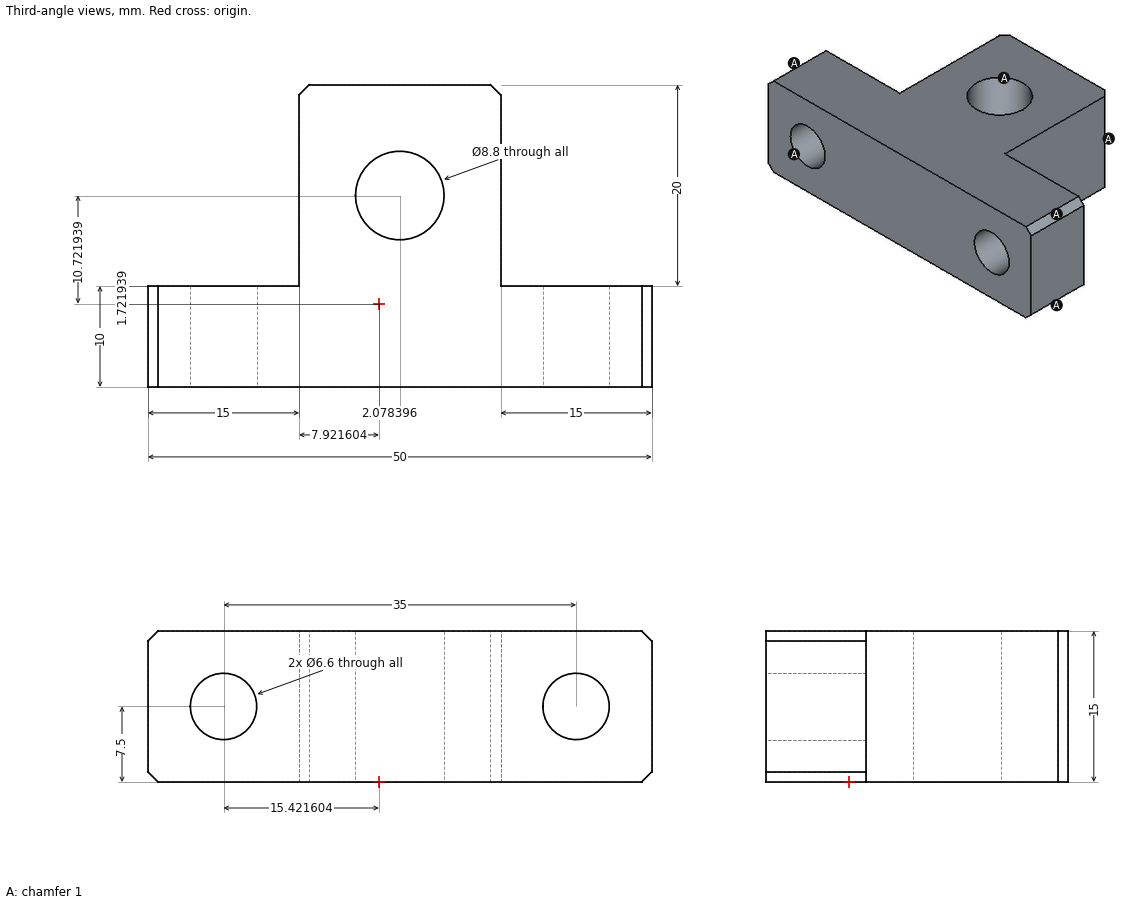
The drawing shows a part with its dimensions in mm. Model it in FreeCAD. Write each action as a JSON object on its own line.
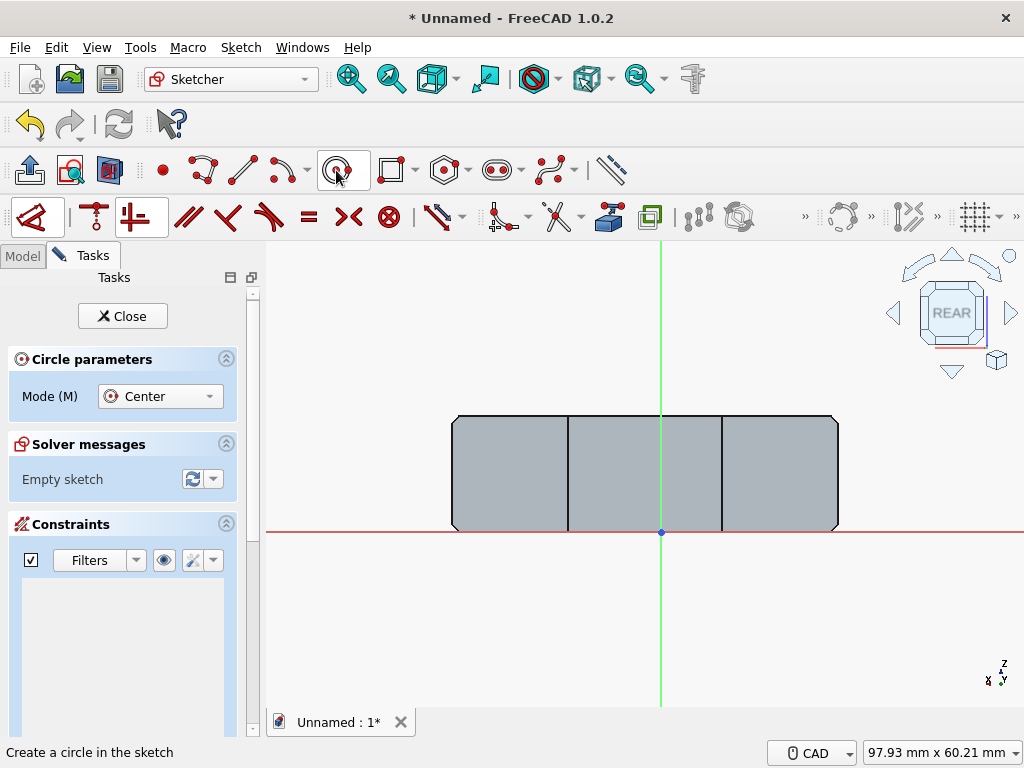
{"action": "left_click", "coordinate": [780, 474]}
{"action": "mouse_move", "coordinate": [799, 456]}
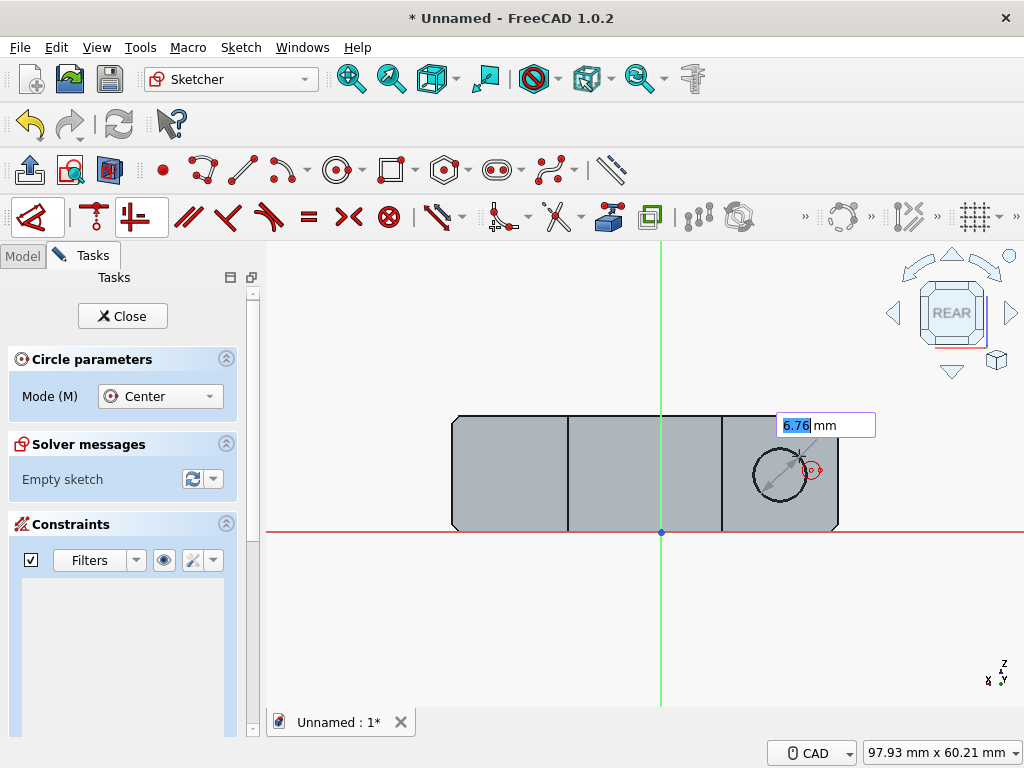
{"action": "type", "text": "6.6"}
{"action": "key", "text": "Return"}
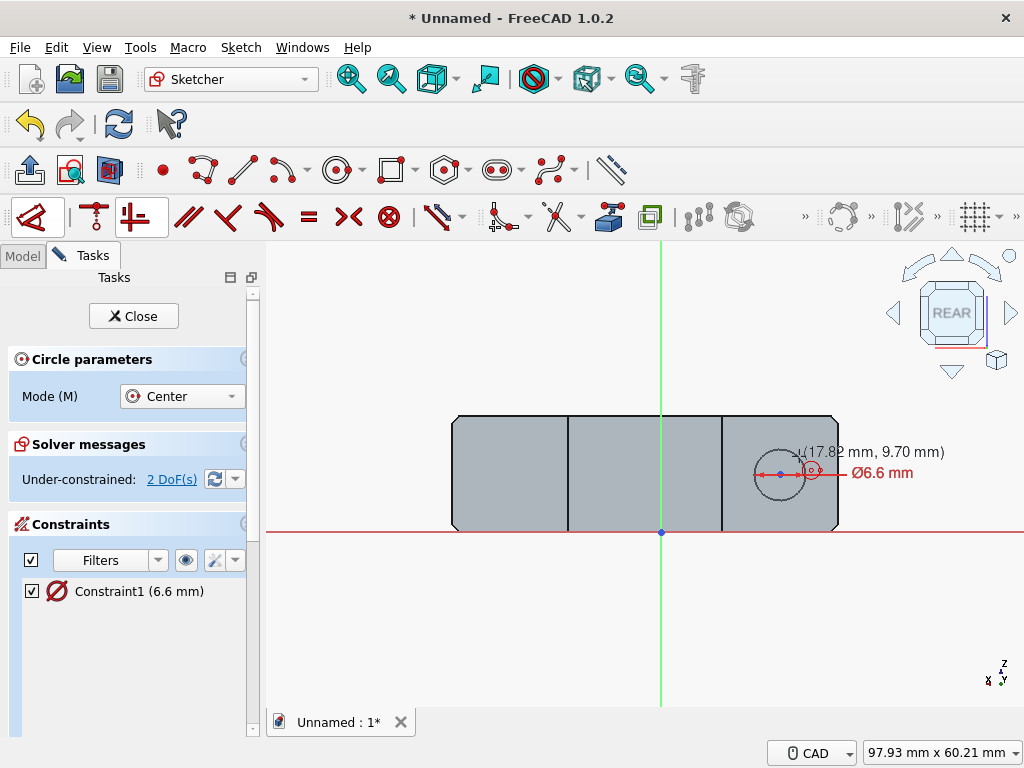
{"action": "left_click", "coordinate": [510, 474]}
{"action": "mouse_move", "coordinate": [528, 456]}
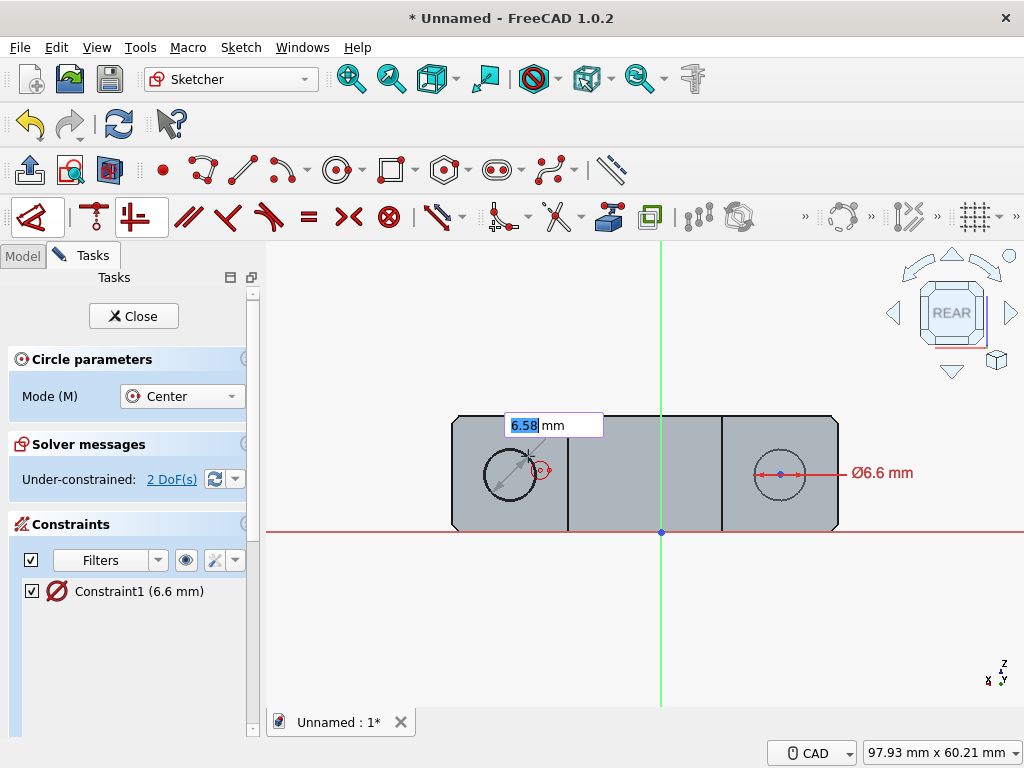
{"action": "type", "text": "6.6"}
{"action": "key", "text": "Return"}
{"action": "key", "text": "Escape"}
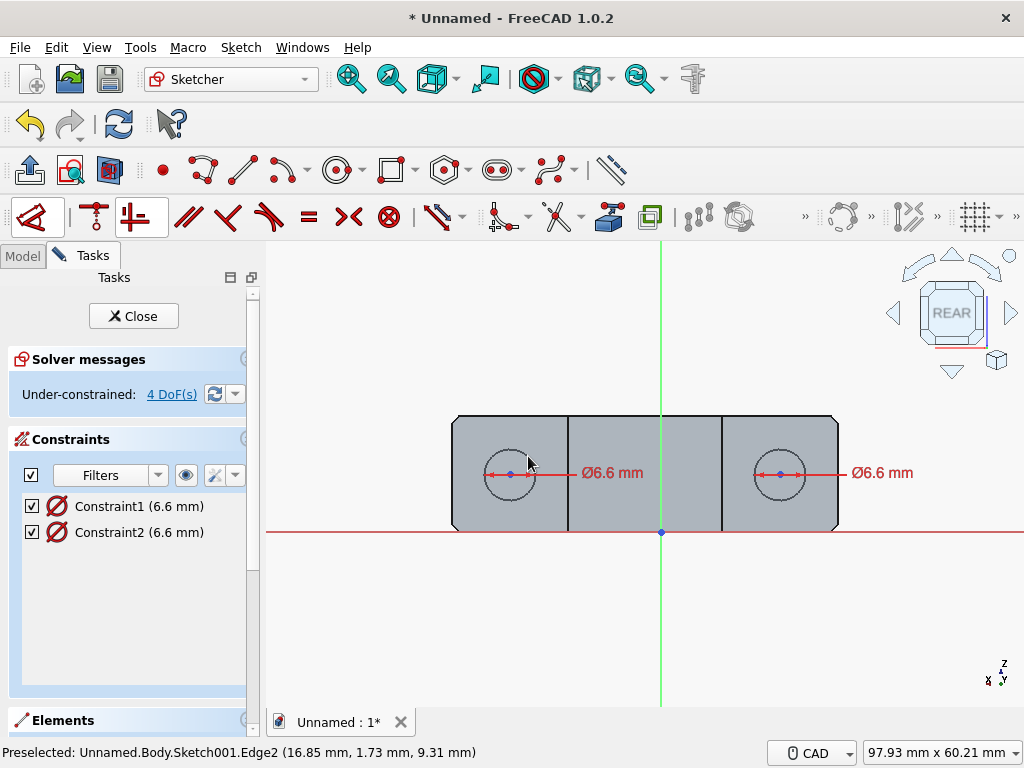
{"action": "left_click", "coordinate": [780, 475]}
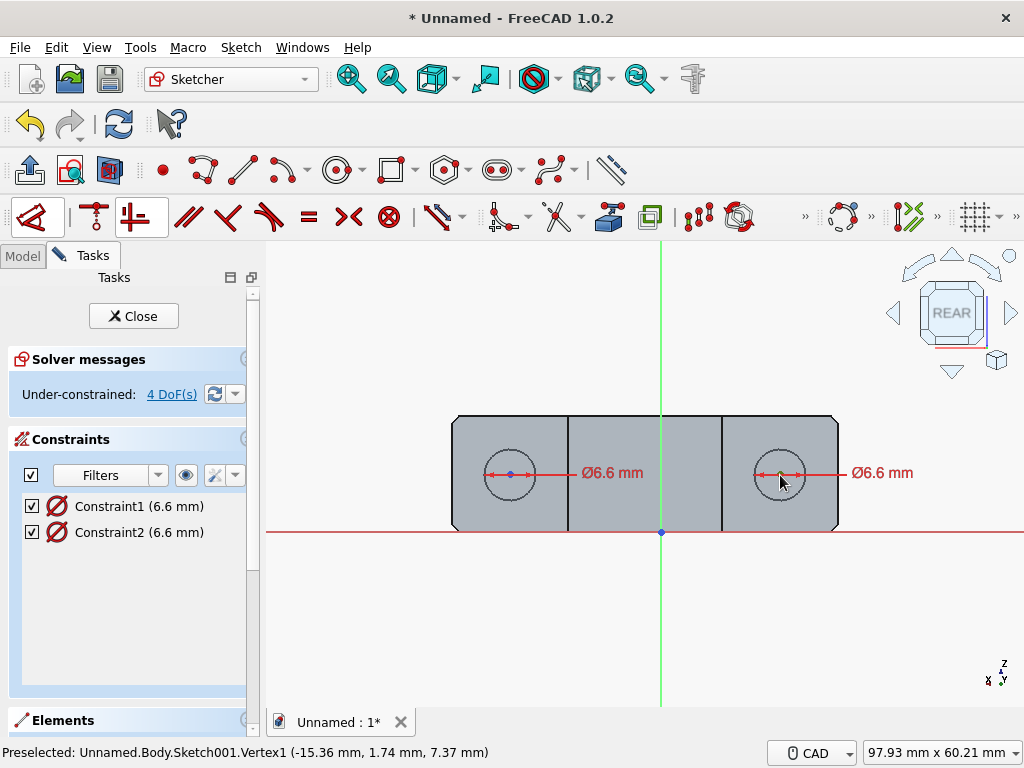
{"action": "left_click", "coordinate": [58, 218]}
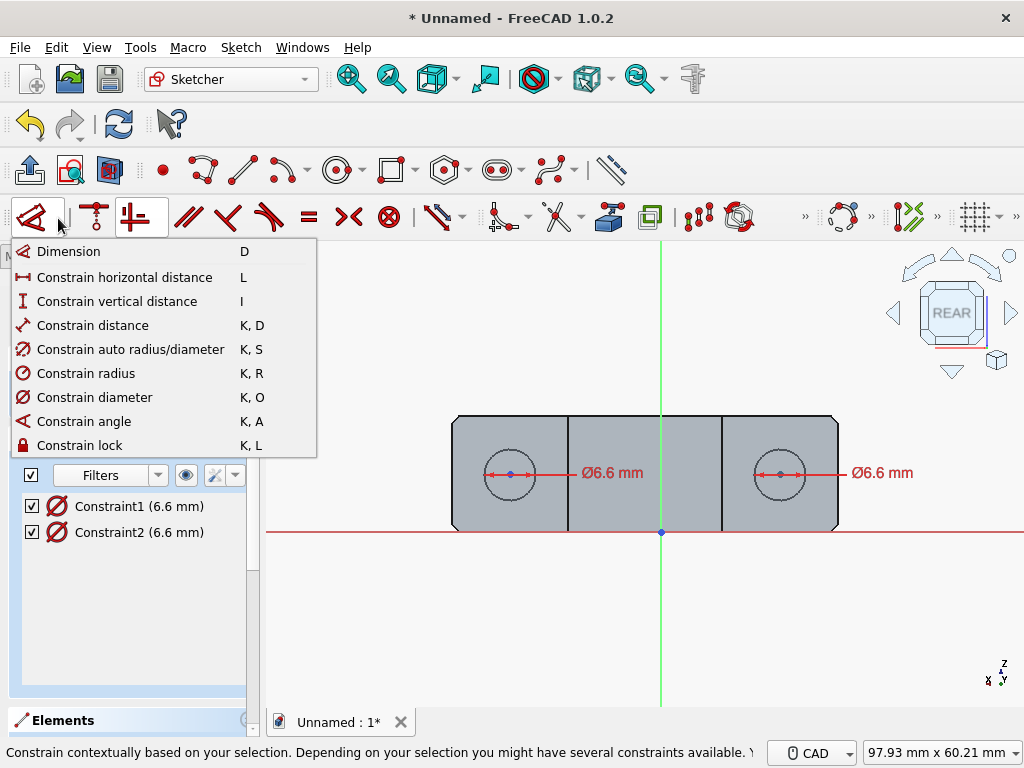
{"action": "left_click", "coordinate": [164, 301]}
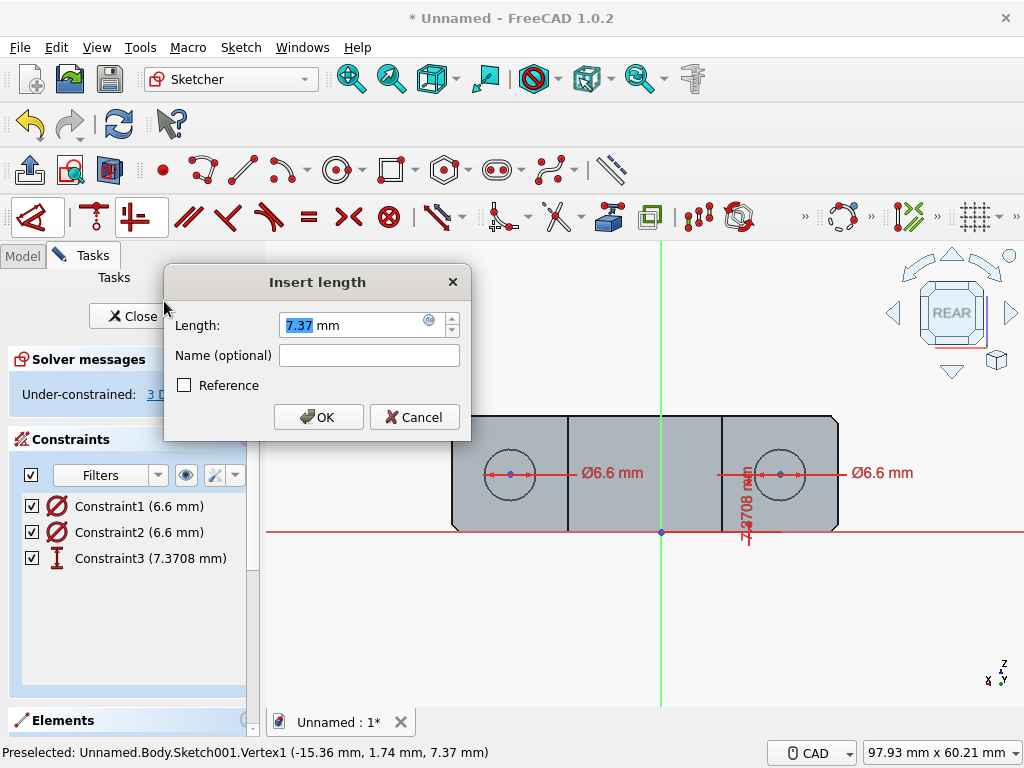
{"action": "type", "text": "7.5"}
{"action": "key", "text": "Return"}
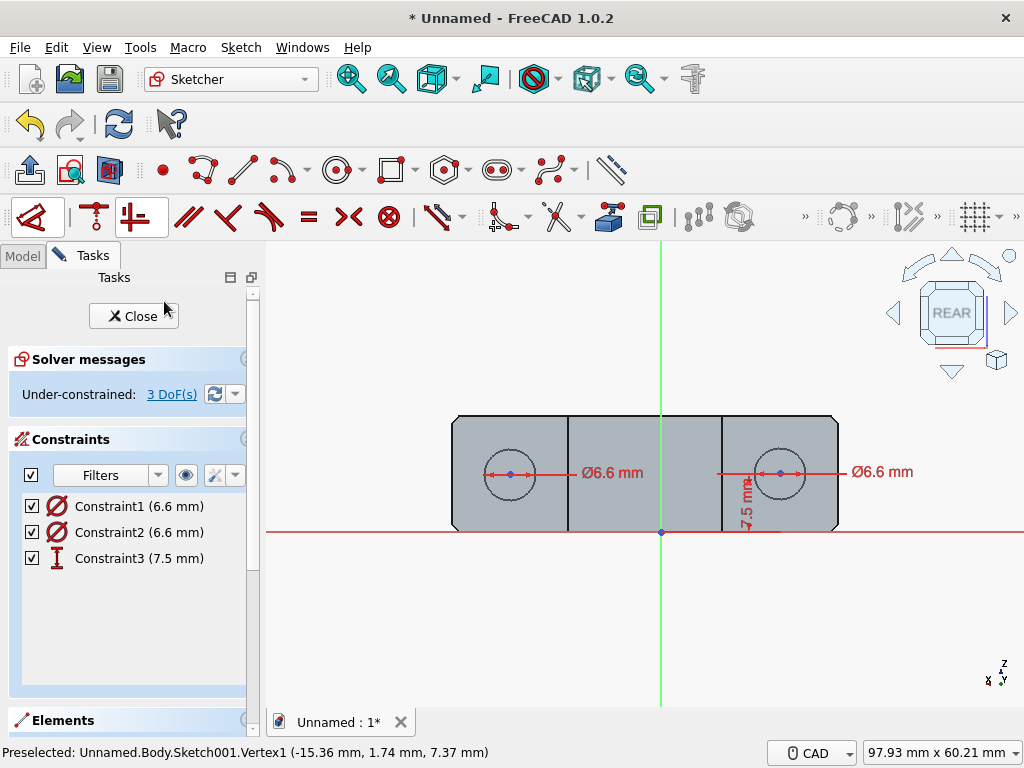
{"action": "left_click", "coordinate": [510, 475]}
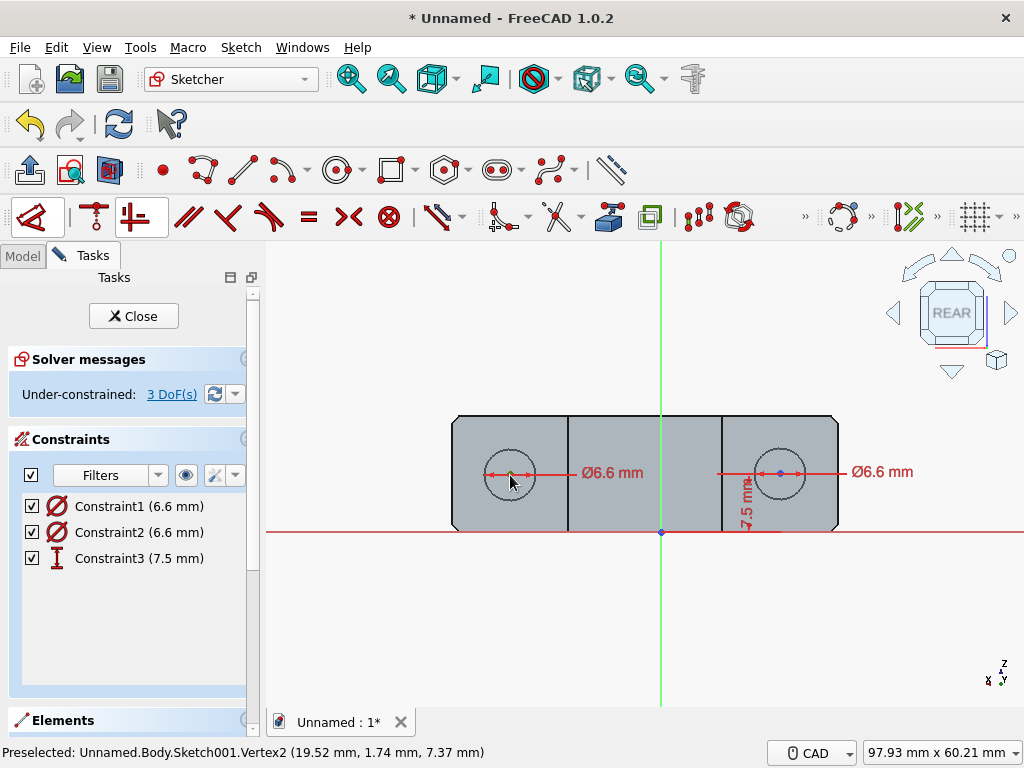
{"action": "left_click", "coordinate": [58, 218]}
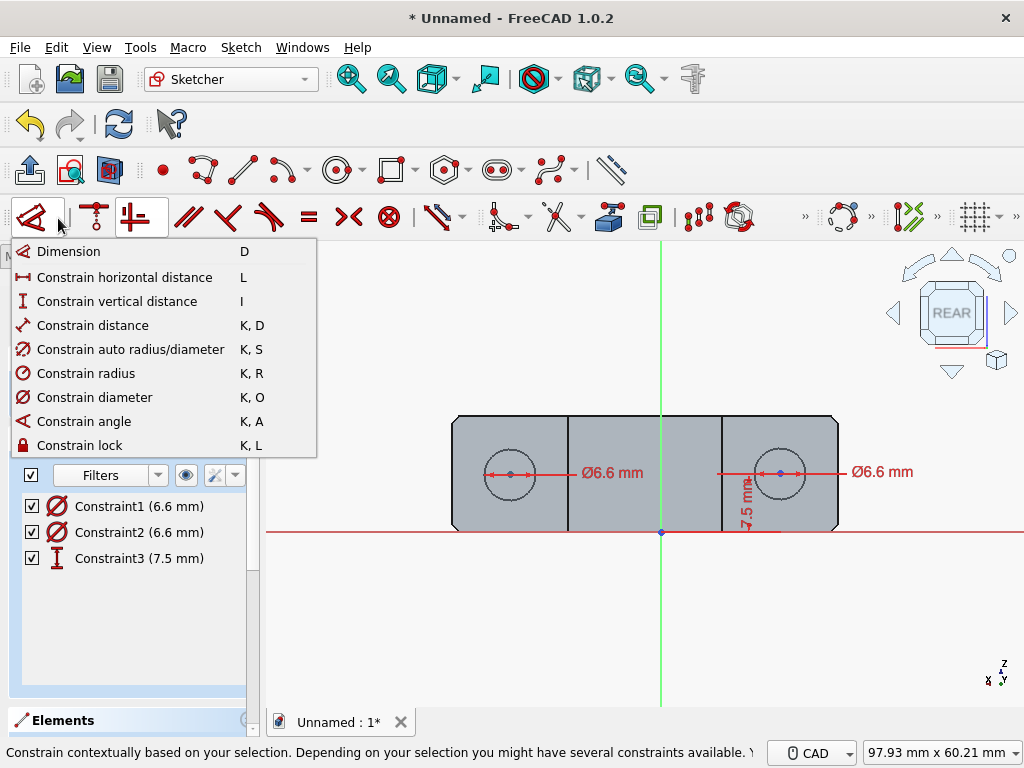
{"action": "left_click", "coordinate": [164, 301]}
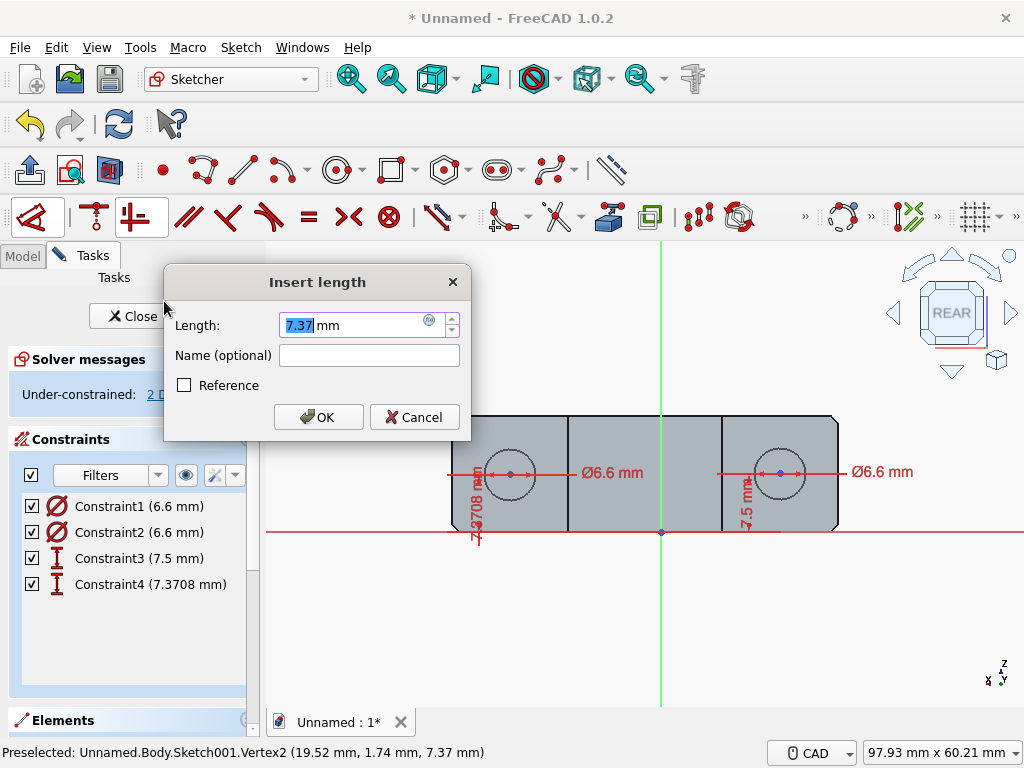
{"action": "type", "text": "7.5"}
{"action": "key", "text": "Return"}